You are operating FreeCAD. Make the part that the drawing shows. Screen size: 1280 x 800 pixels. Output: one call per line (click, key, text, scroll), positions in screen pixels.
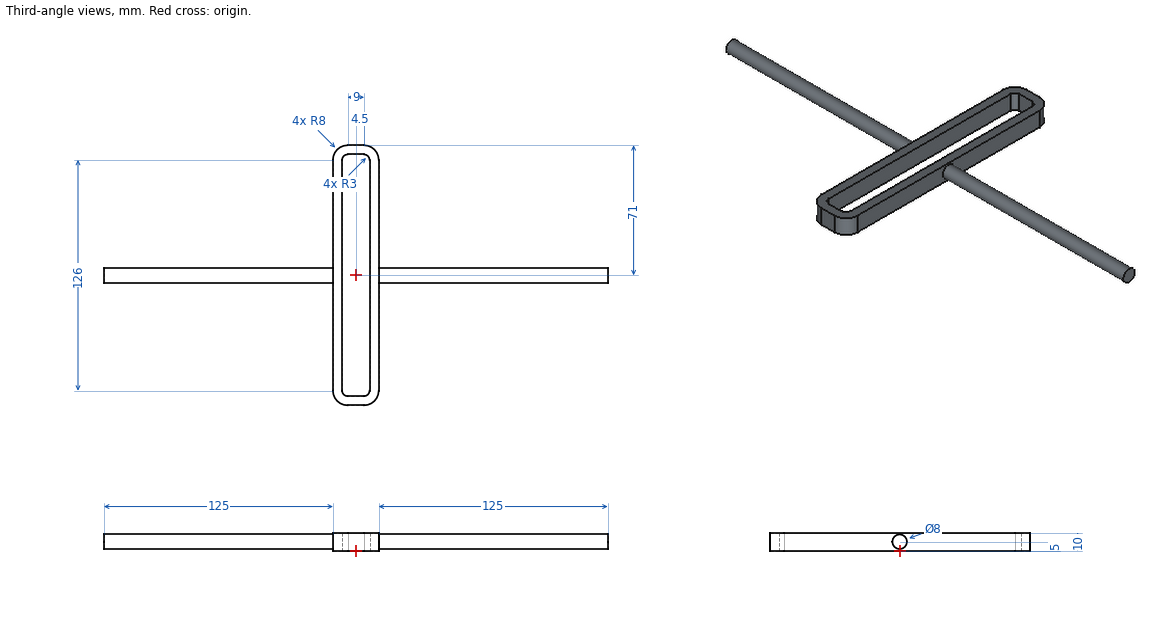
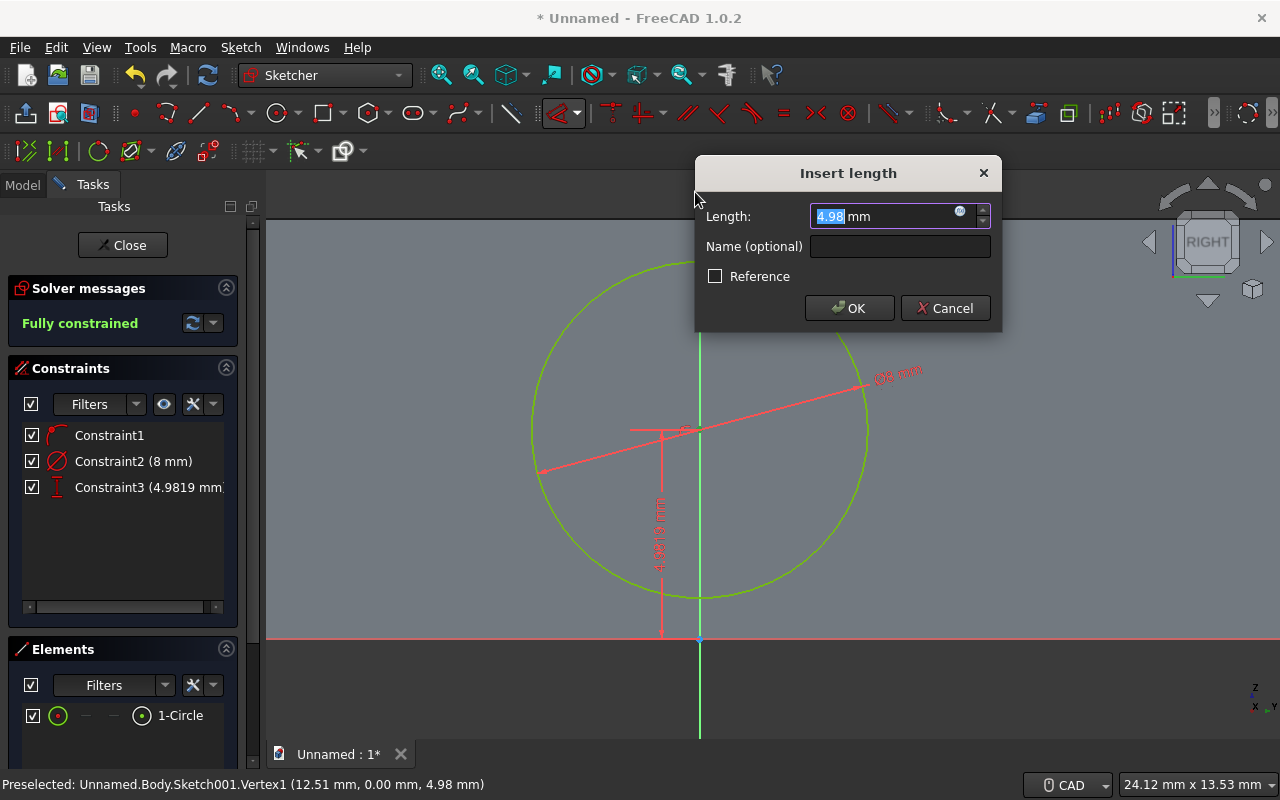
text(5)
key(Return)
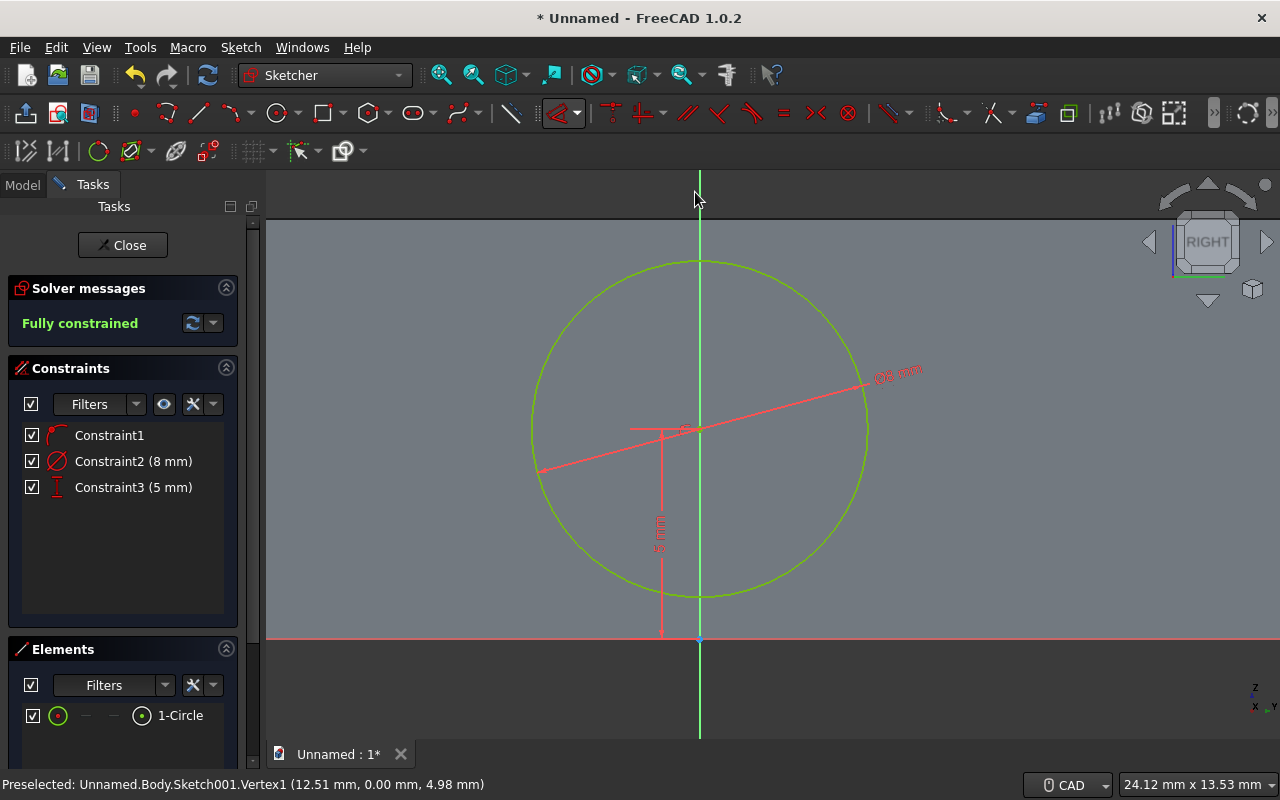
click(123, 245)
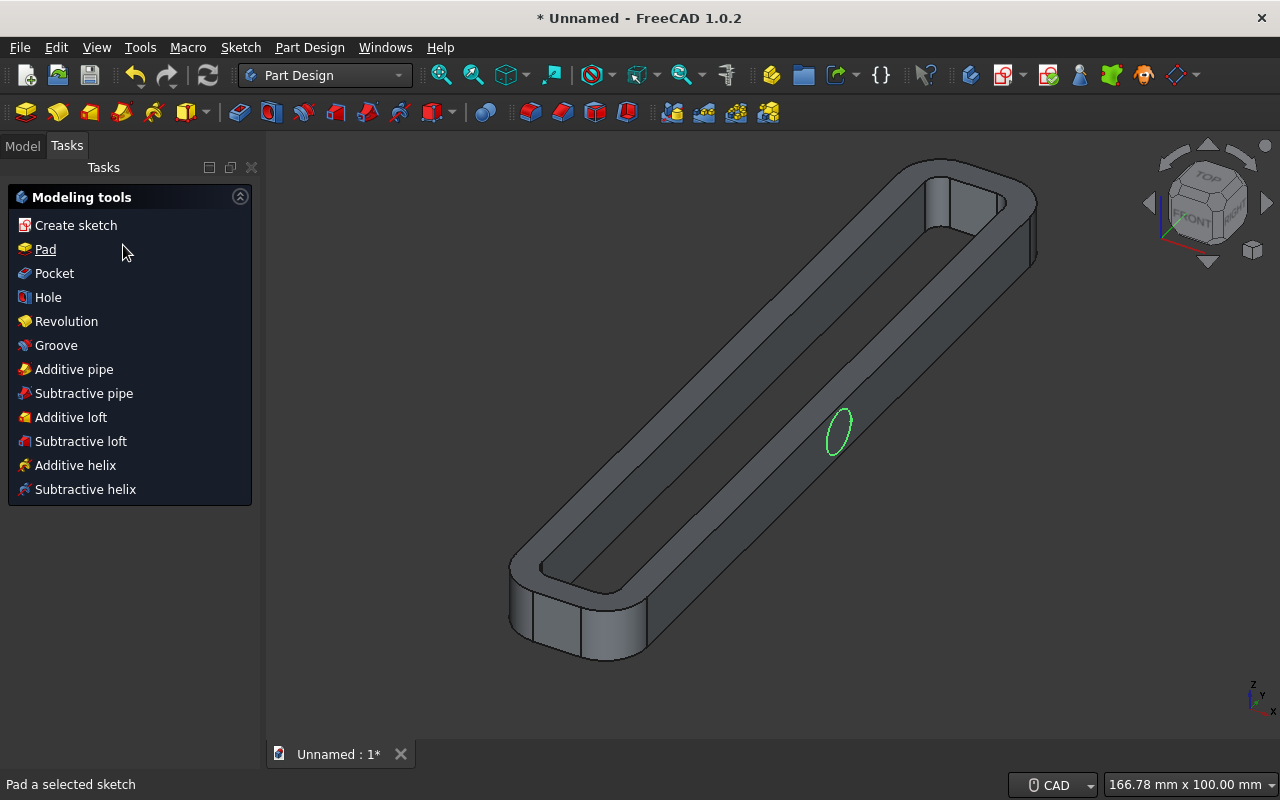
click(26, 112)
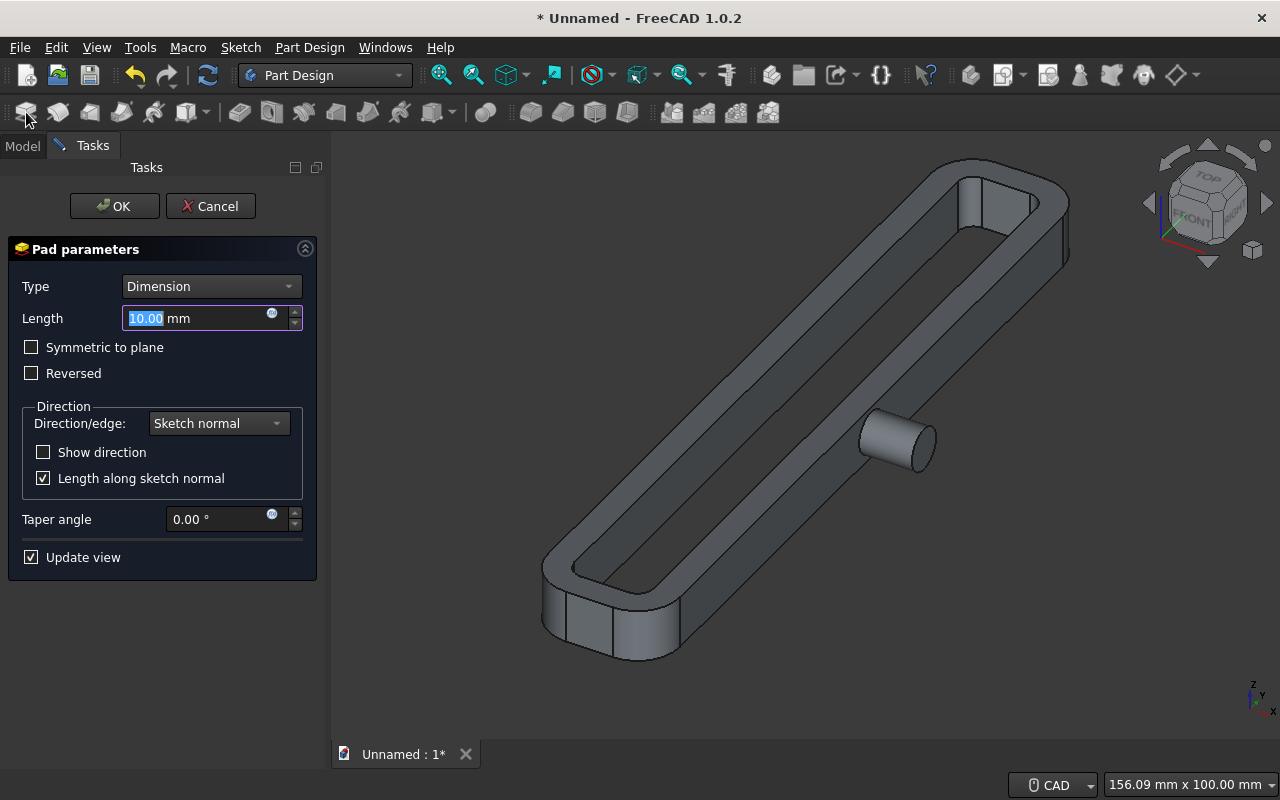
text(125)
key(Tab)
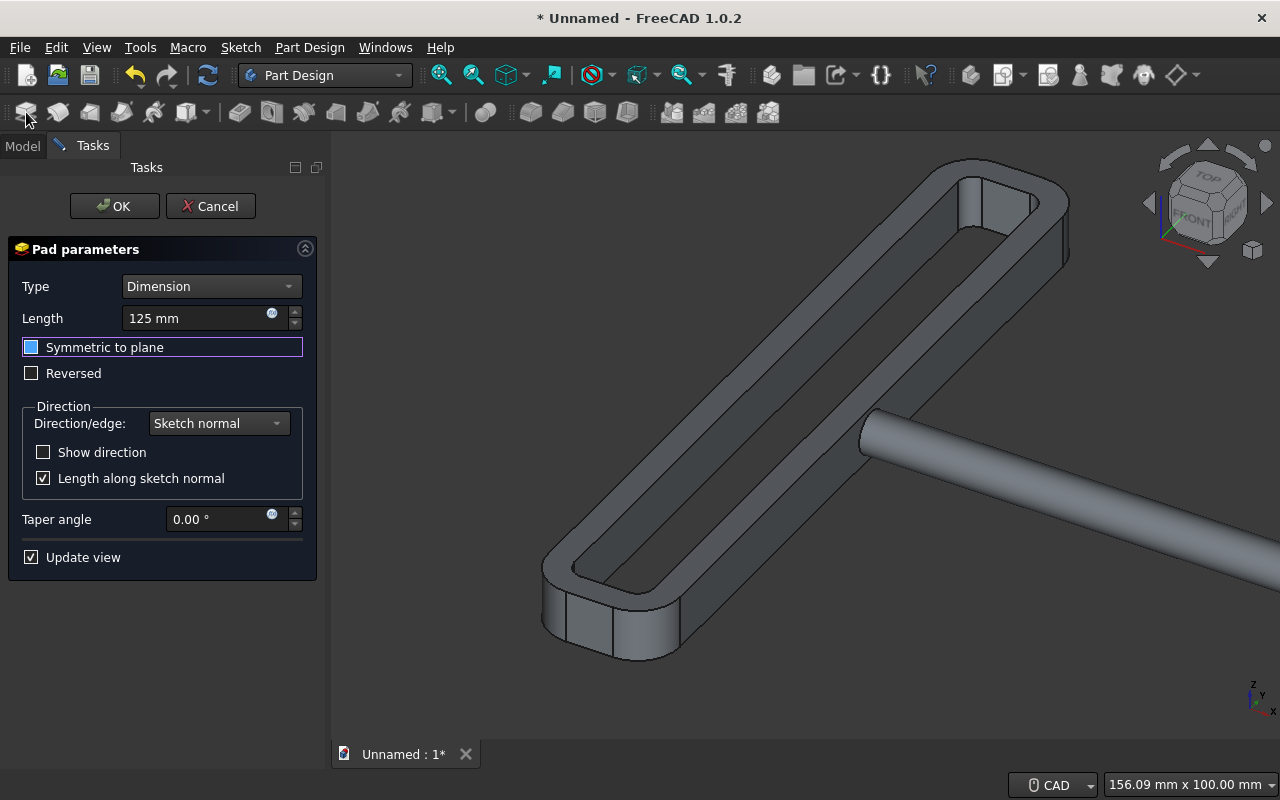
click(115, 206)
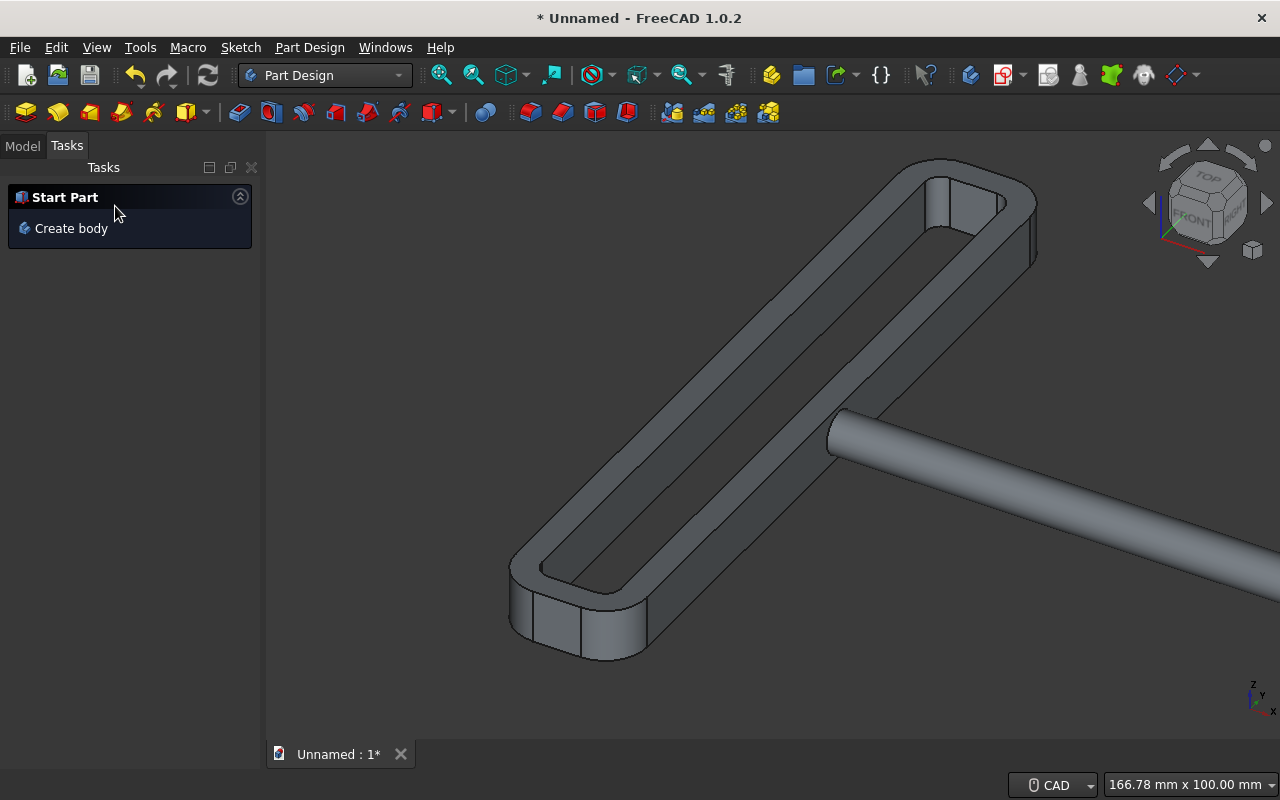
click(442, 76)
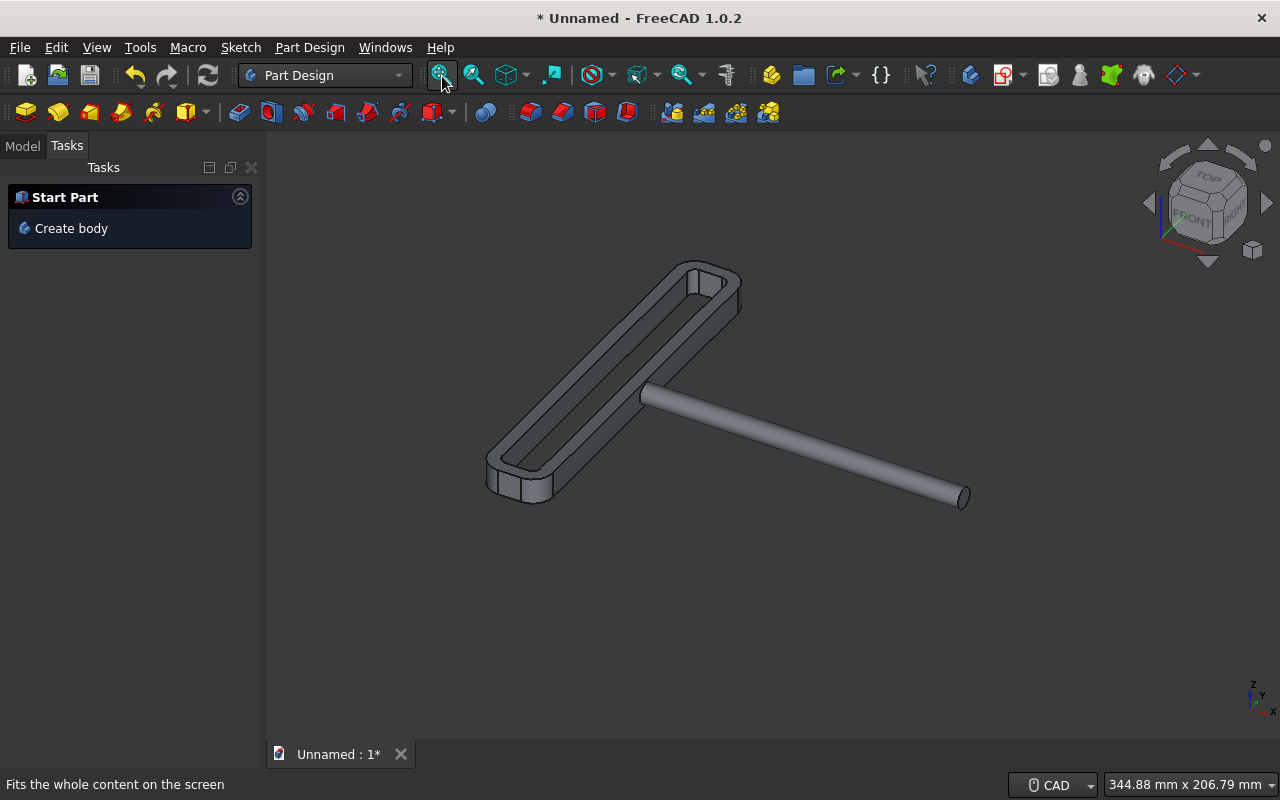
click(23, 145)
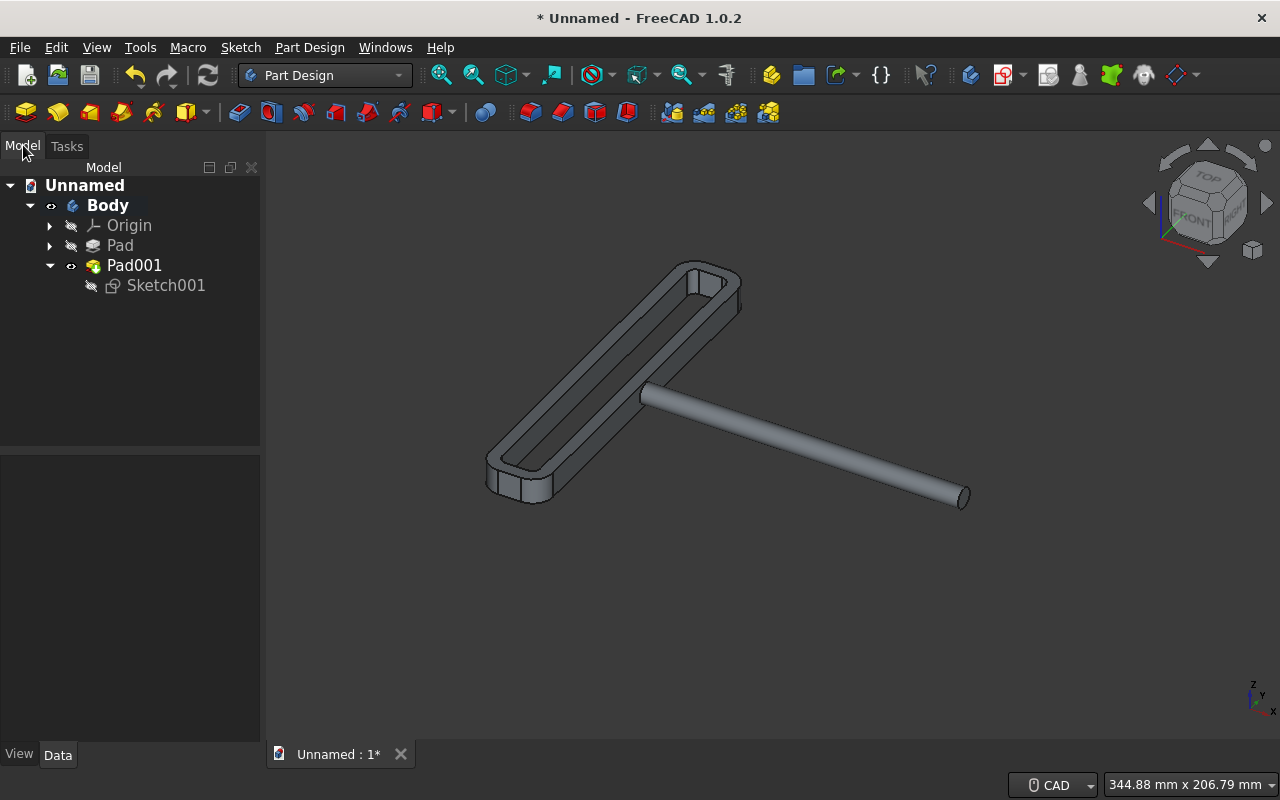
click(50, 226)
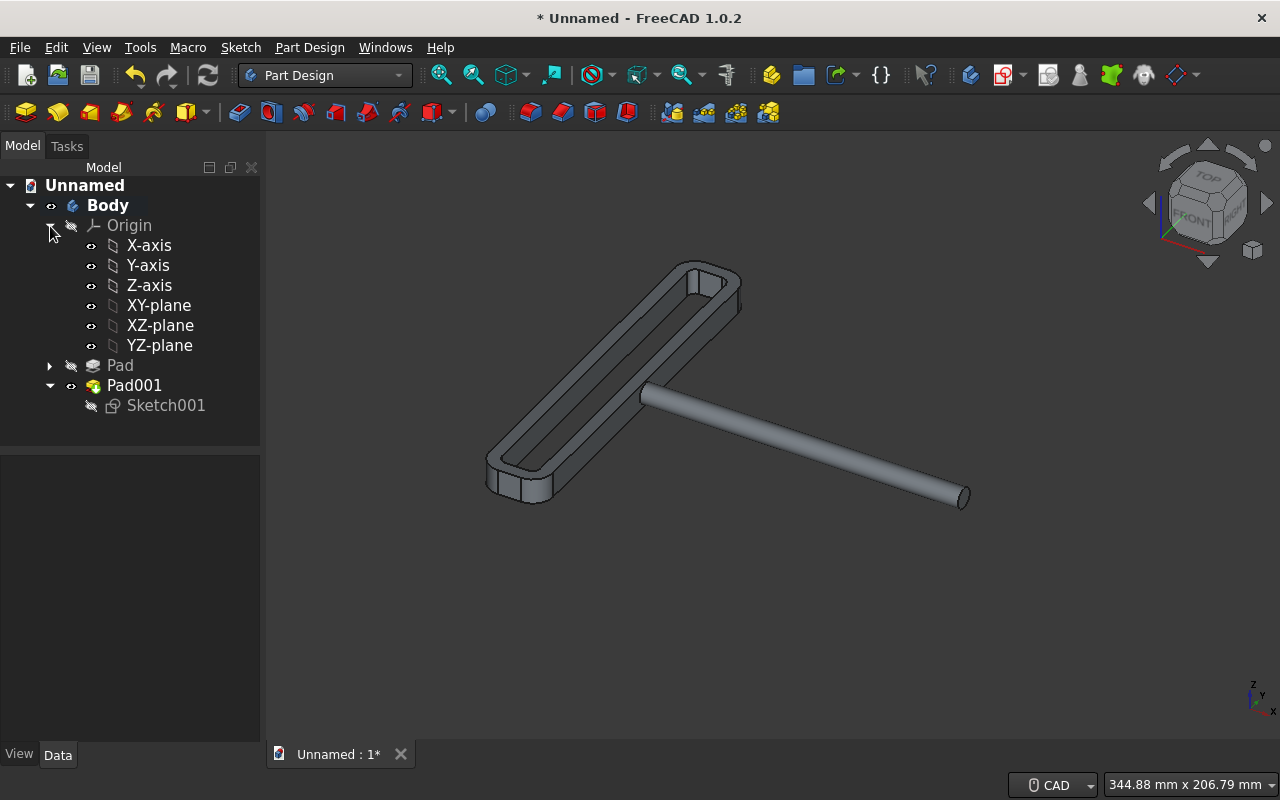
click(136, 346)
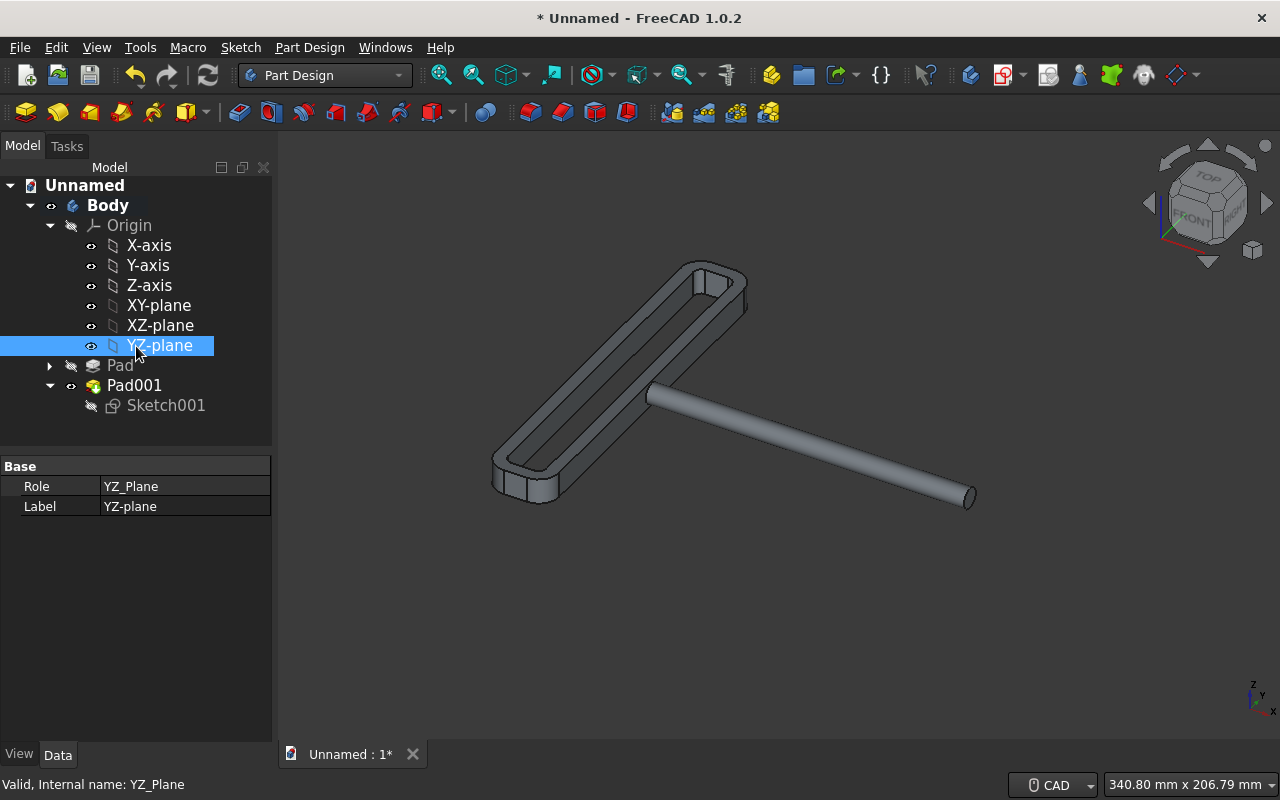
click(1176, 76)